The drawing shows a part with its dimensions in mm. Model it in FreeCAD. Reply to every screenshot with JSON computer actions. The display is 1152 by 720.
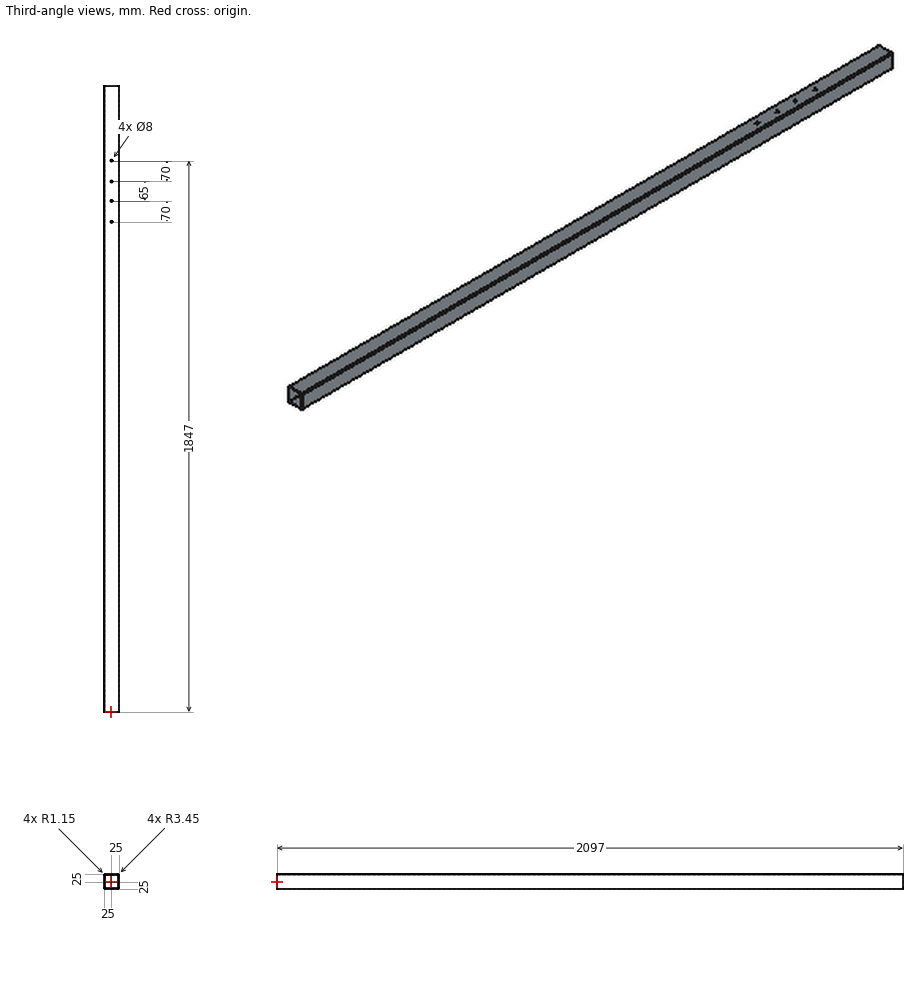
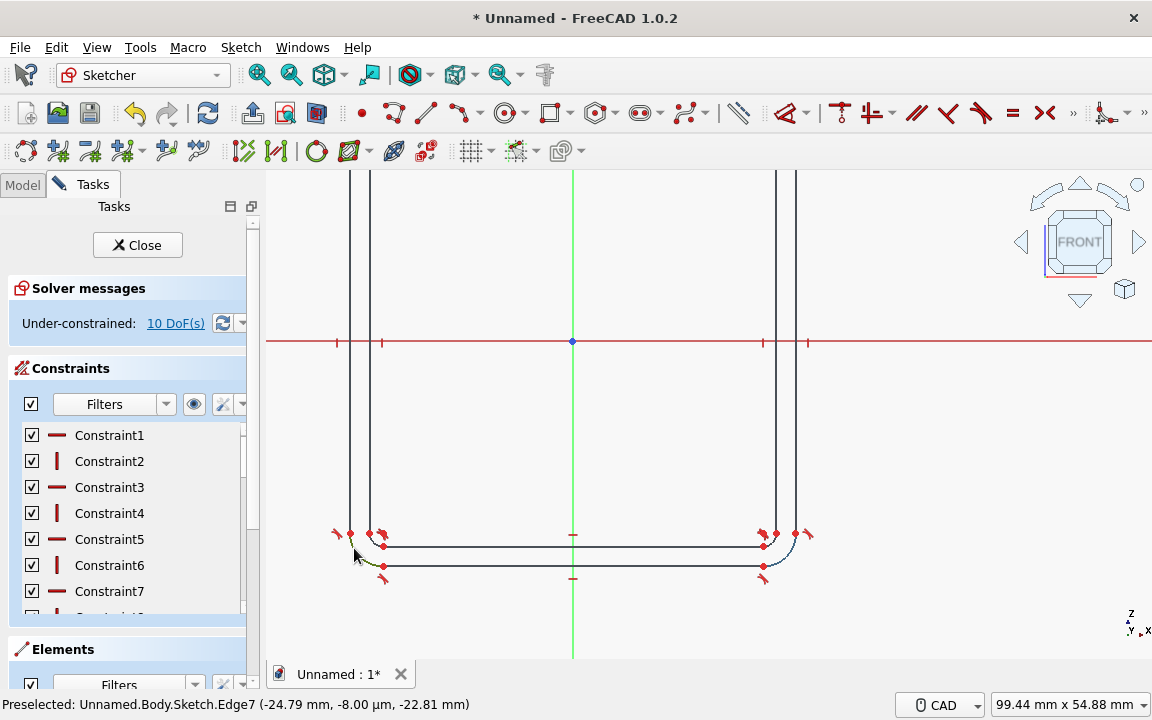
{"action": "scroll", "coordinate": [778, 563], "scroll_direction": "down", "scroll_amount": 2}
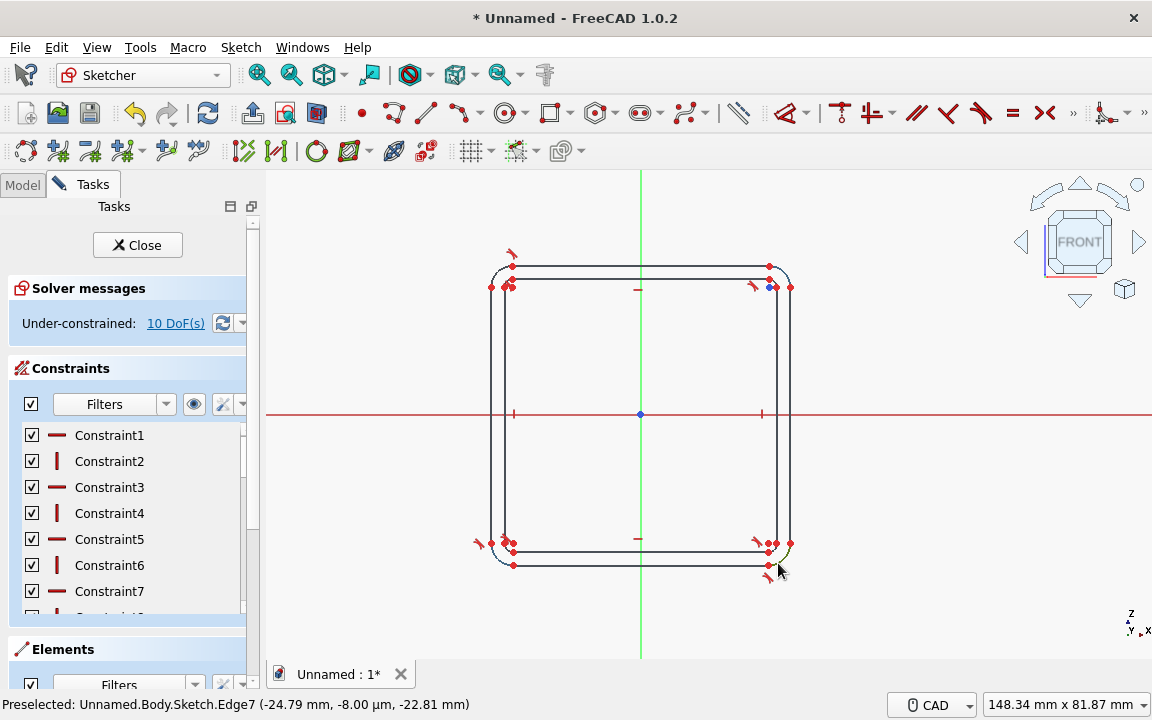
{"action": "scroll", "coordinate": [503, 268], "scroll_direction": "up", "scroll_amount": 2}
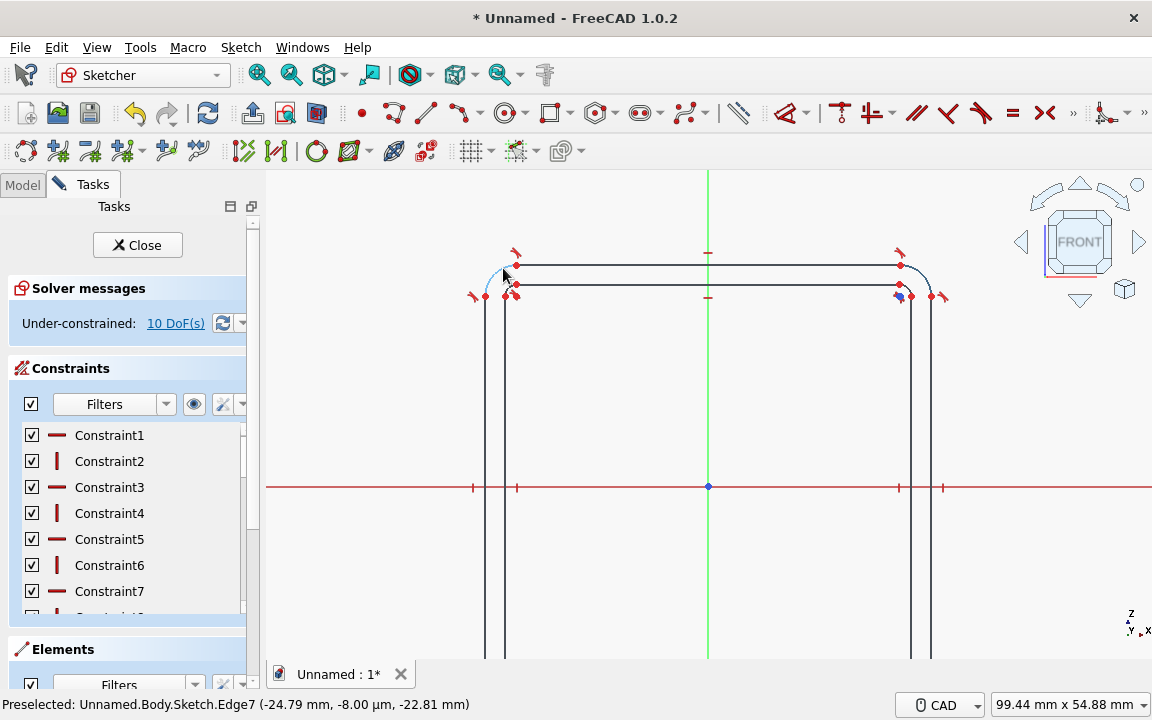
{"action": "left_click", "coordinate": [502, 269]}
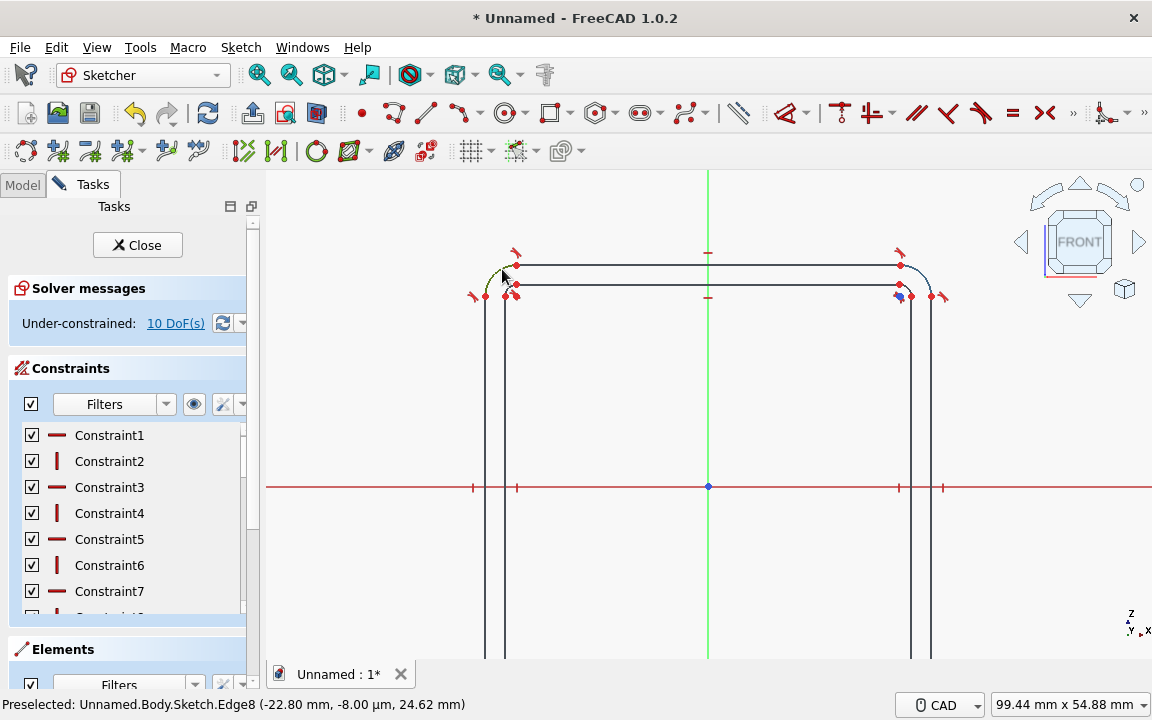
{"action": "left_click", "coordinate": [1014, 114]}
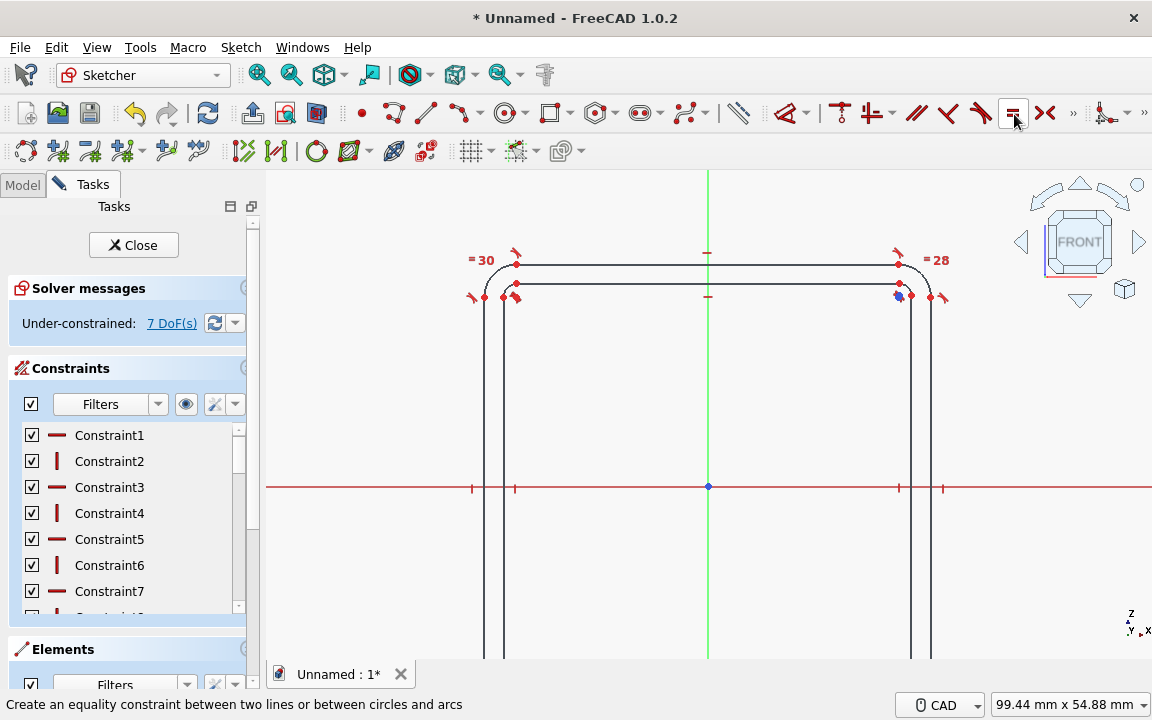
{"action": "scroll", "coordinate": [508, 288], "scroll_direction": "up", "scroll_amount": 2}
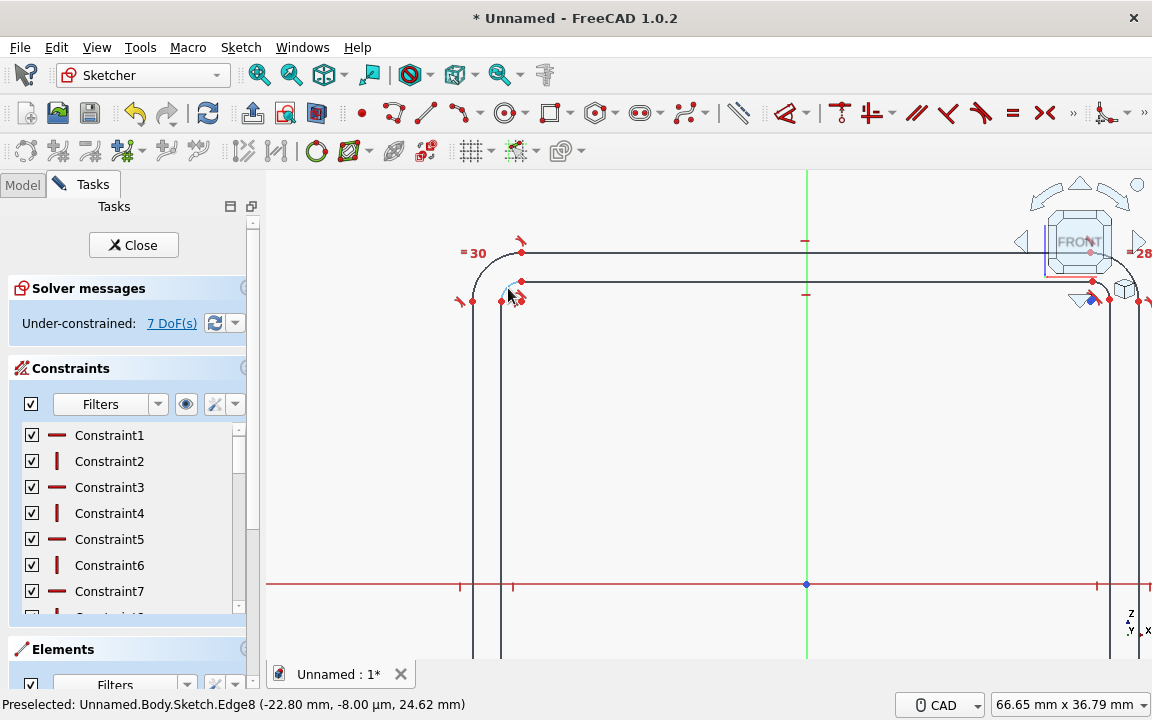
{"action": "left_click", "coordinate": [507, 288]}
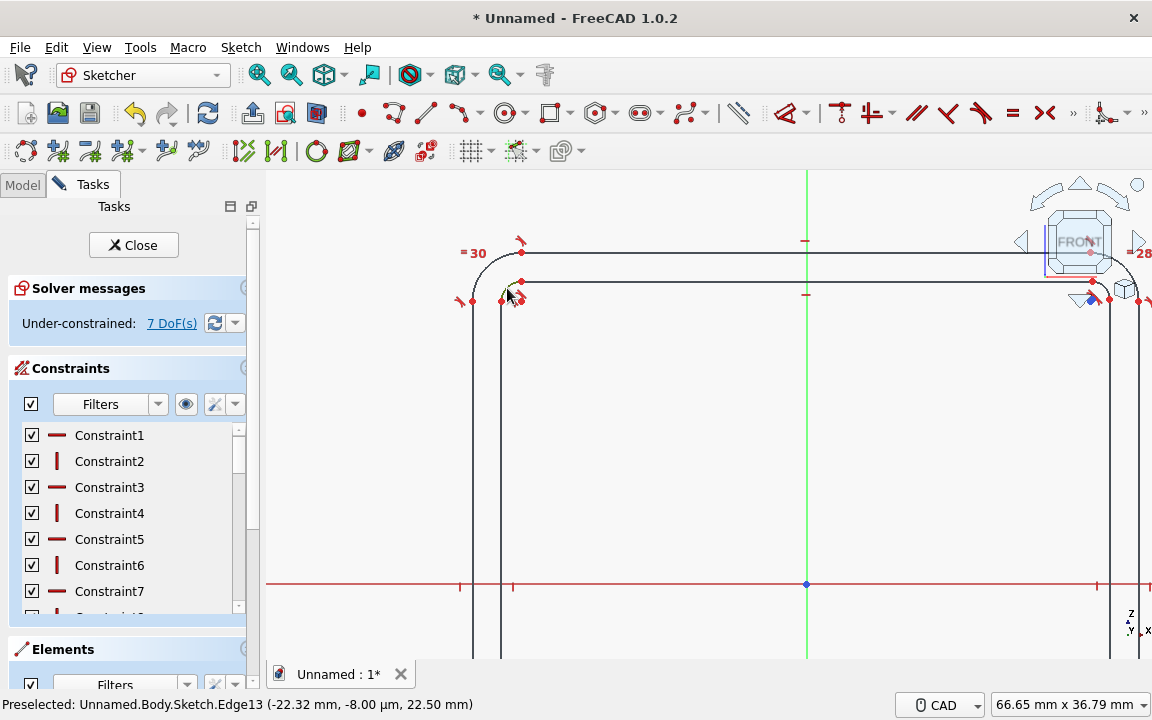
{"action": "scroll", "coordinate": [505, 276], "scroll_direction": "down", "scroll_amount": 4}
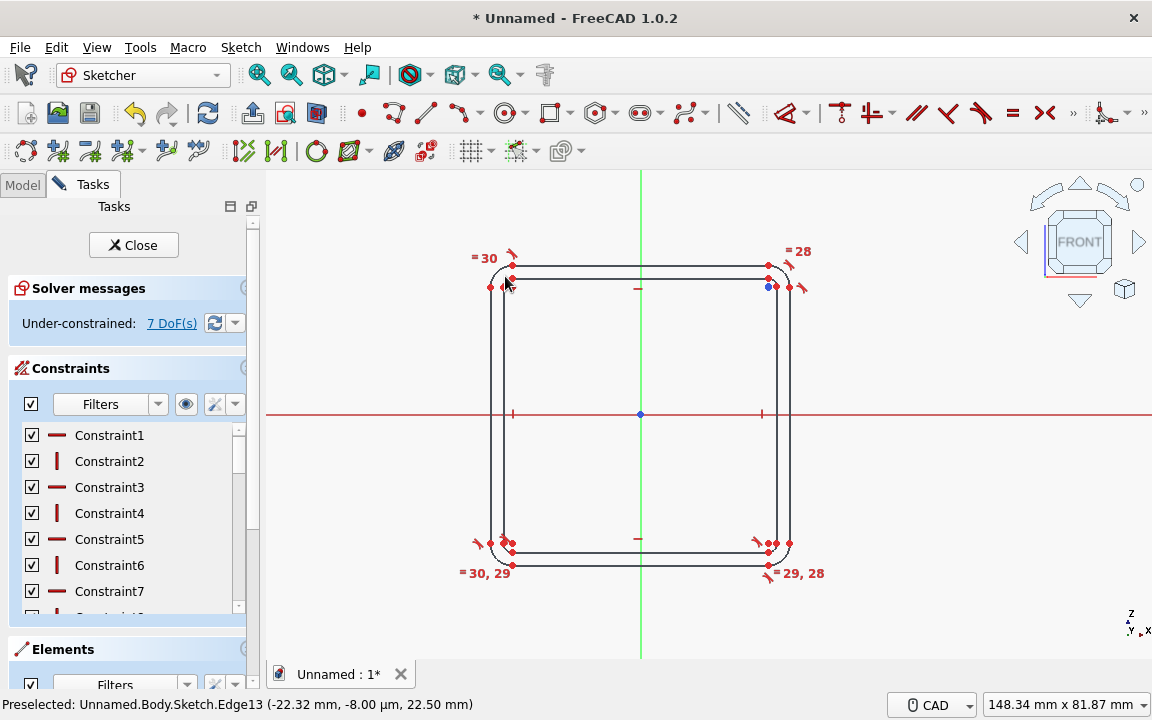
{"action": "scroll", "coordinate": [775, 281], "scroll_direction": "up", "scroll_amount": 5}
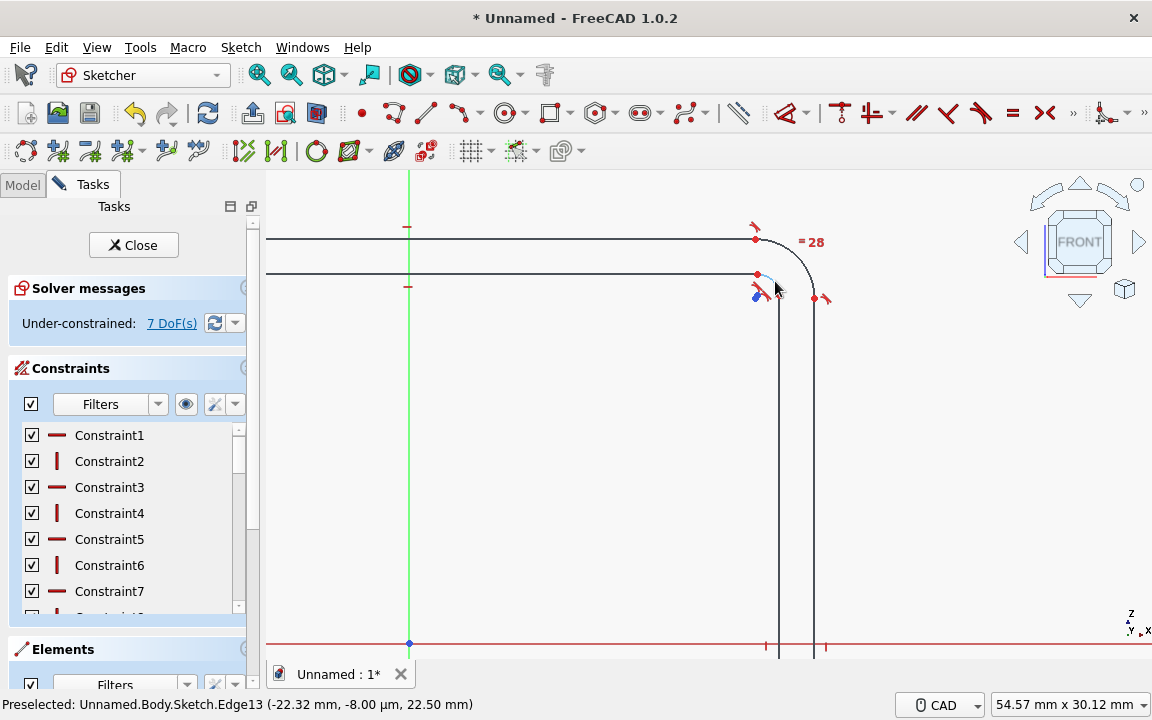
{"action": "left_click", "coordinate": [773, 281]}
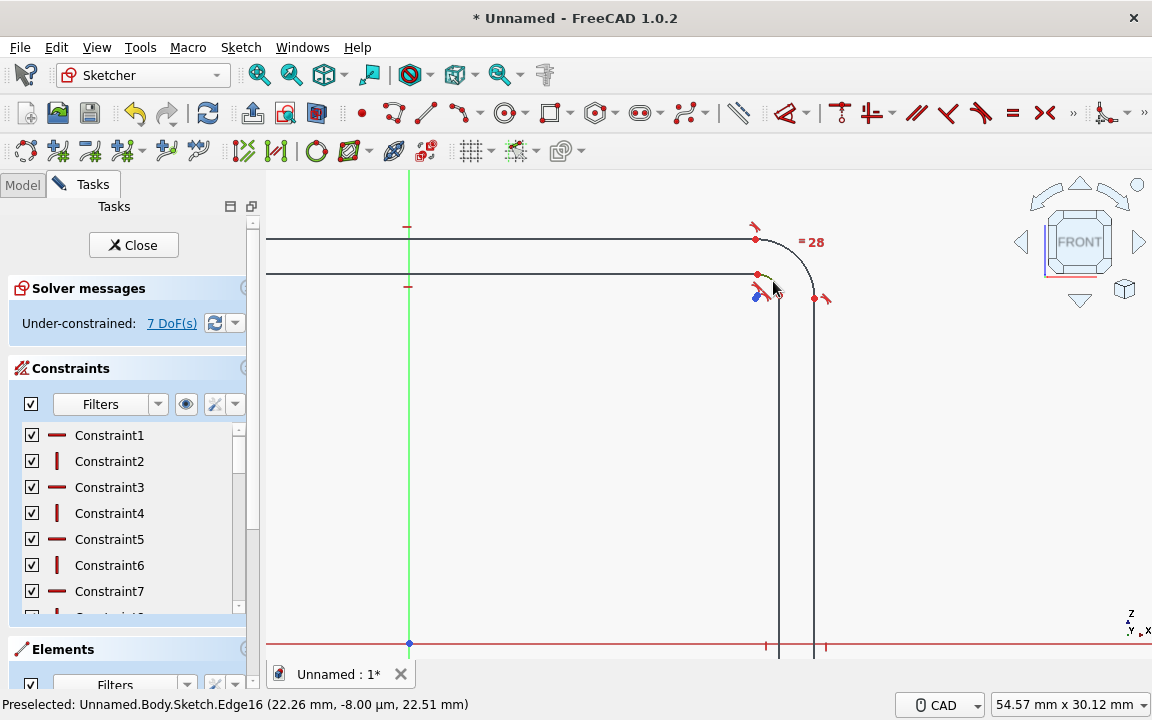
{"action": "left_click", "coordinate": [1014, 114]}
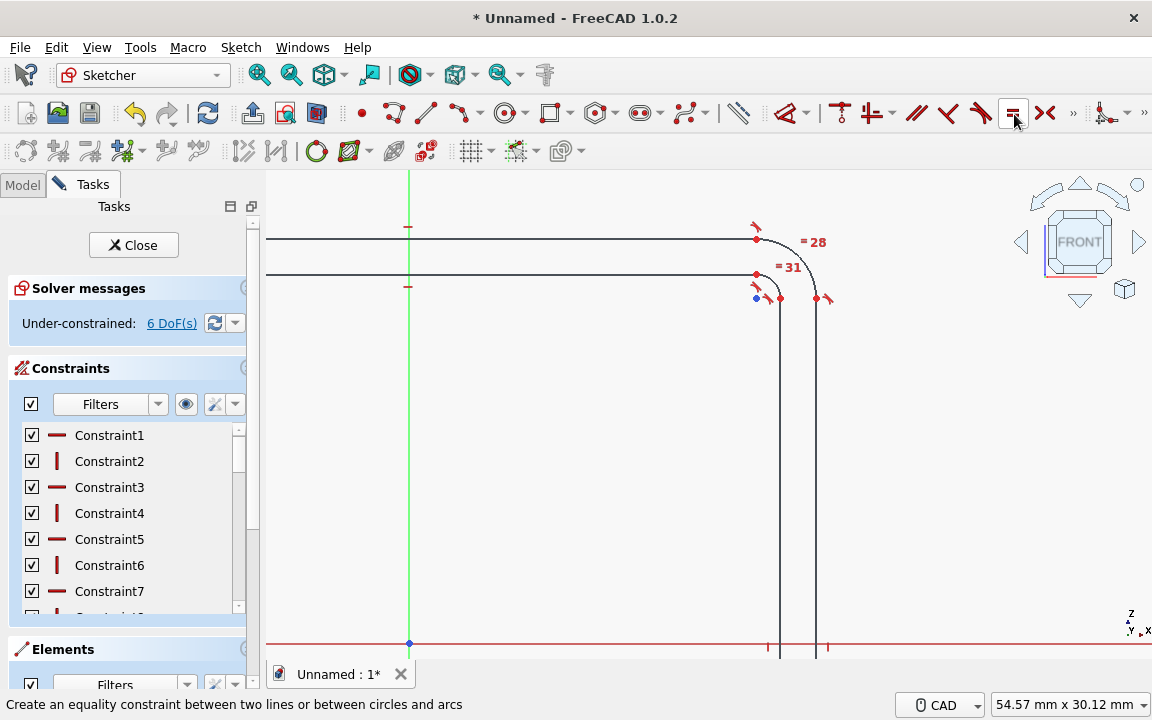
{"action": "left_click", "coordinate": [786, 114]}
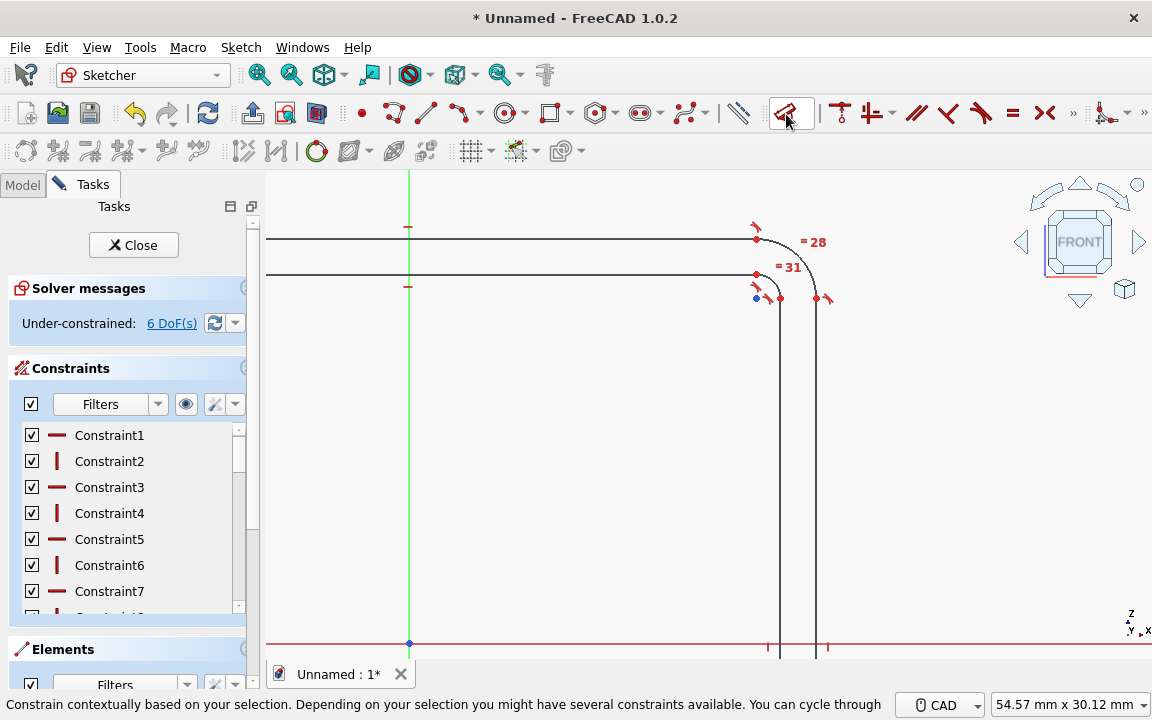
{"action": "left_click", "coordinate": [810, 272]}
{"action": "left_click", "coordinate": [839, 258]}